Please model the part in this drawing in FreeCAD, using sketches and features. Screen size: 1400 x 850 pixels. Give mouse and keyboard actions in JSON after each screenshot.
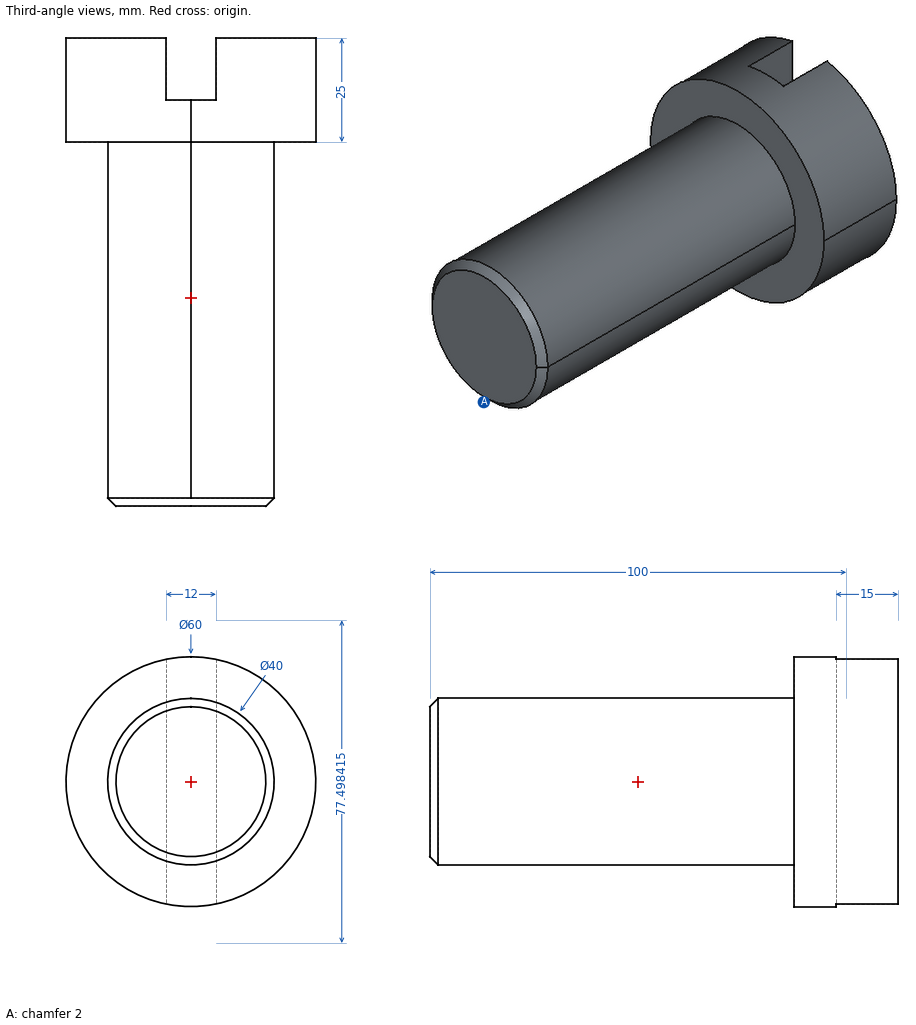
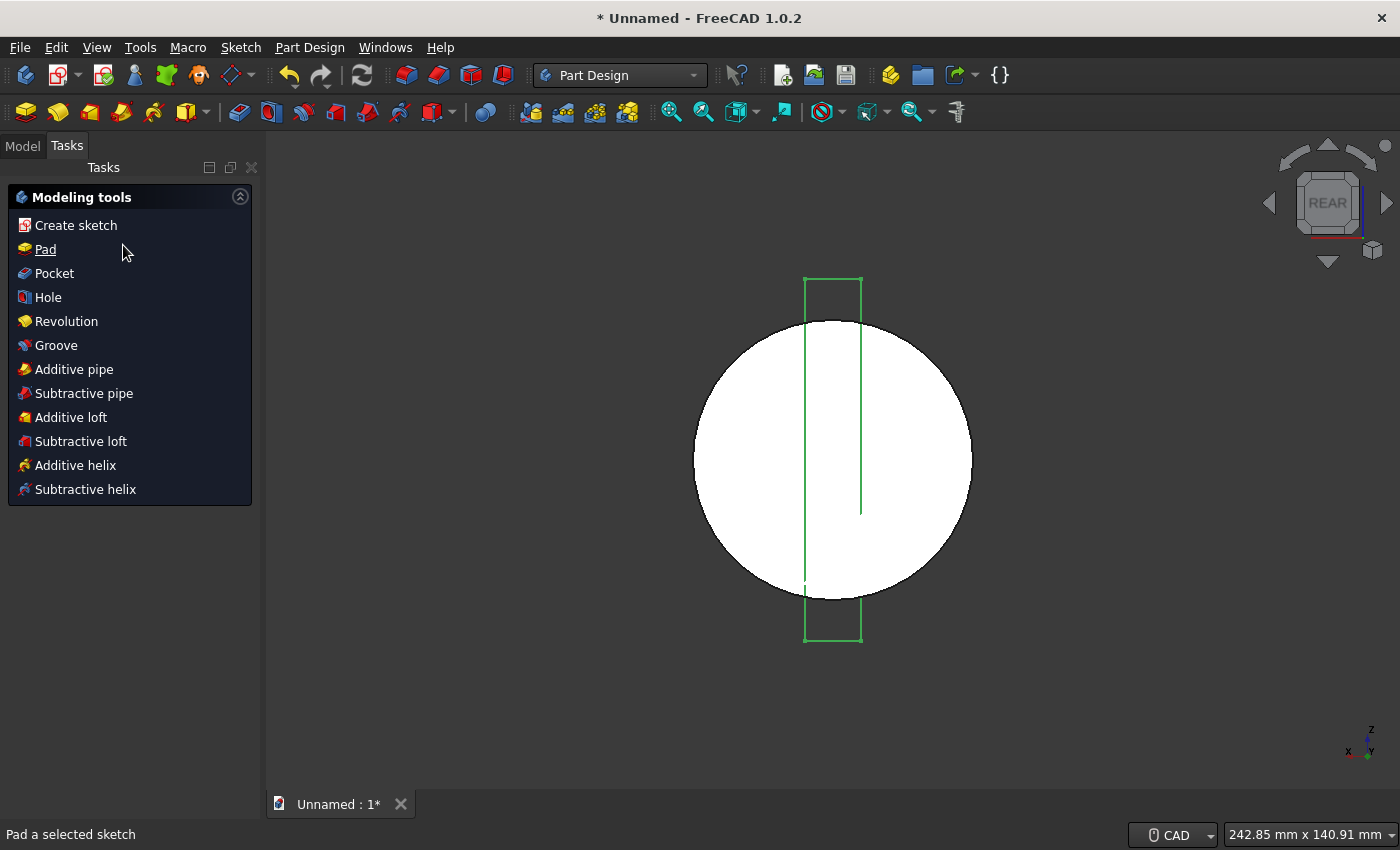
{"action": "left_click", "coordinate": [240, 112]}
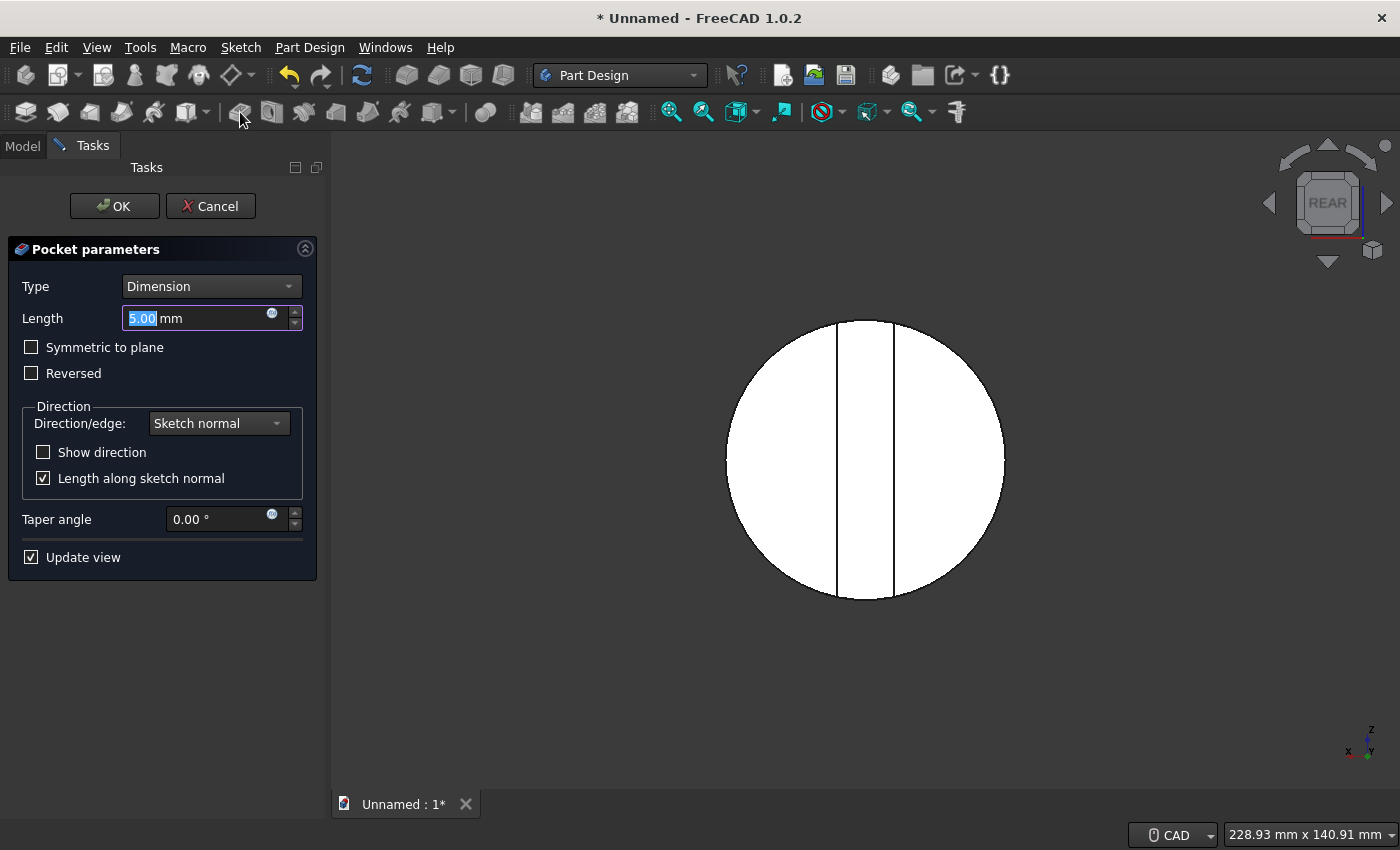
{"action": "type", "text": "15"}
{"action": "key", "text": "Tab"}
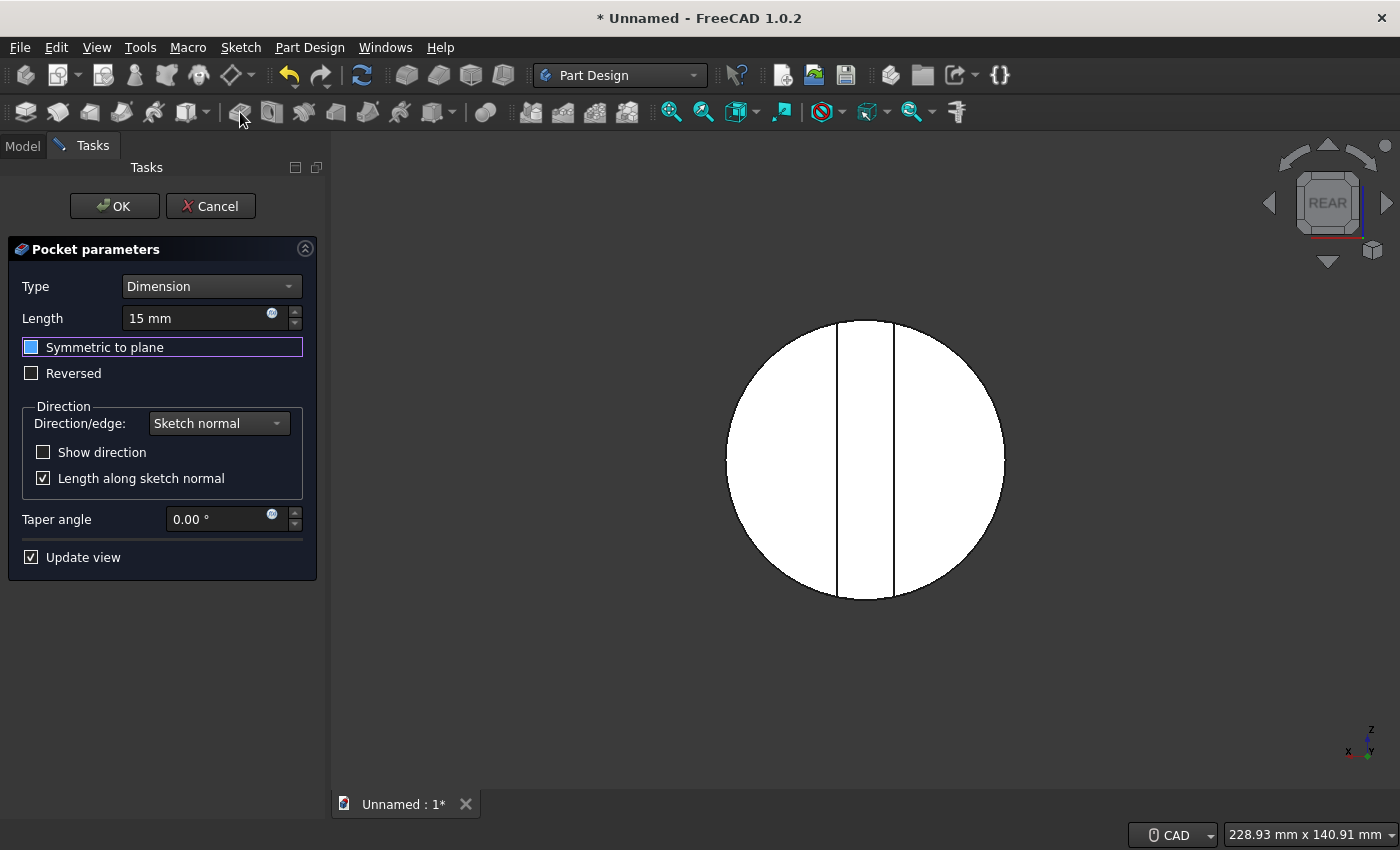
{"action": "left_click", "coordinate": [115, 206]}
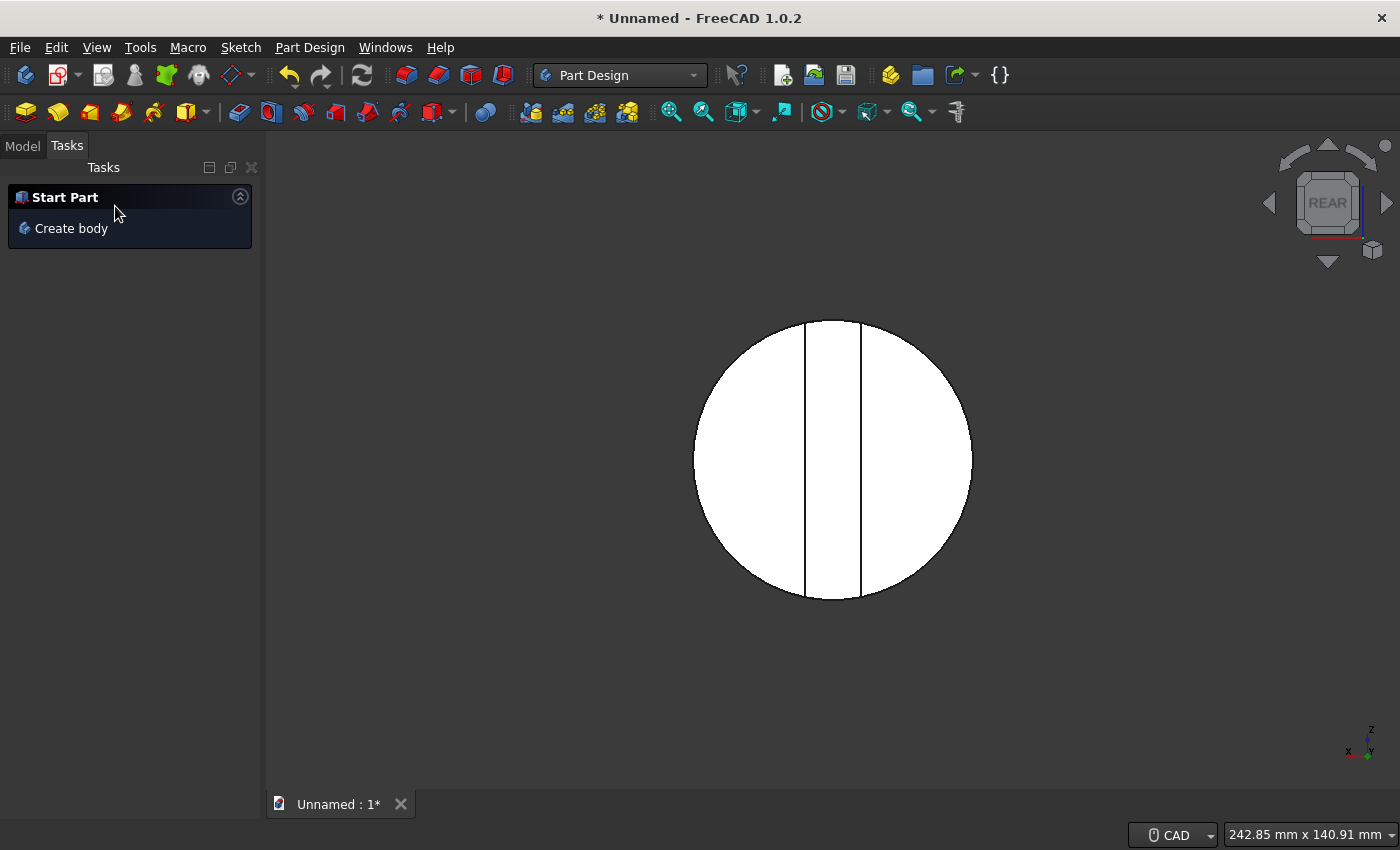
{"action": "key", "text": "0"}